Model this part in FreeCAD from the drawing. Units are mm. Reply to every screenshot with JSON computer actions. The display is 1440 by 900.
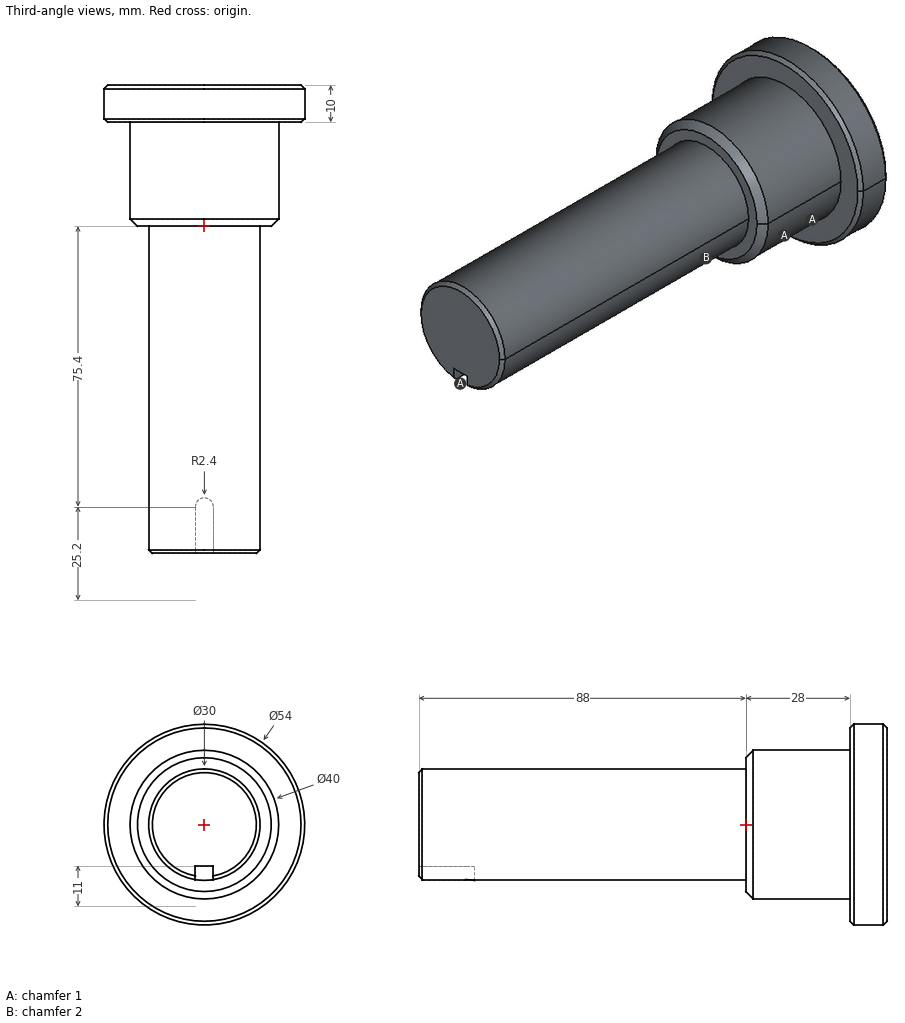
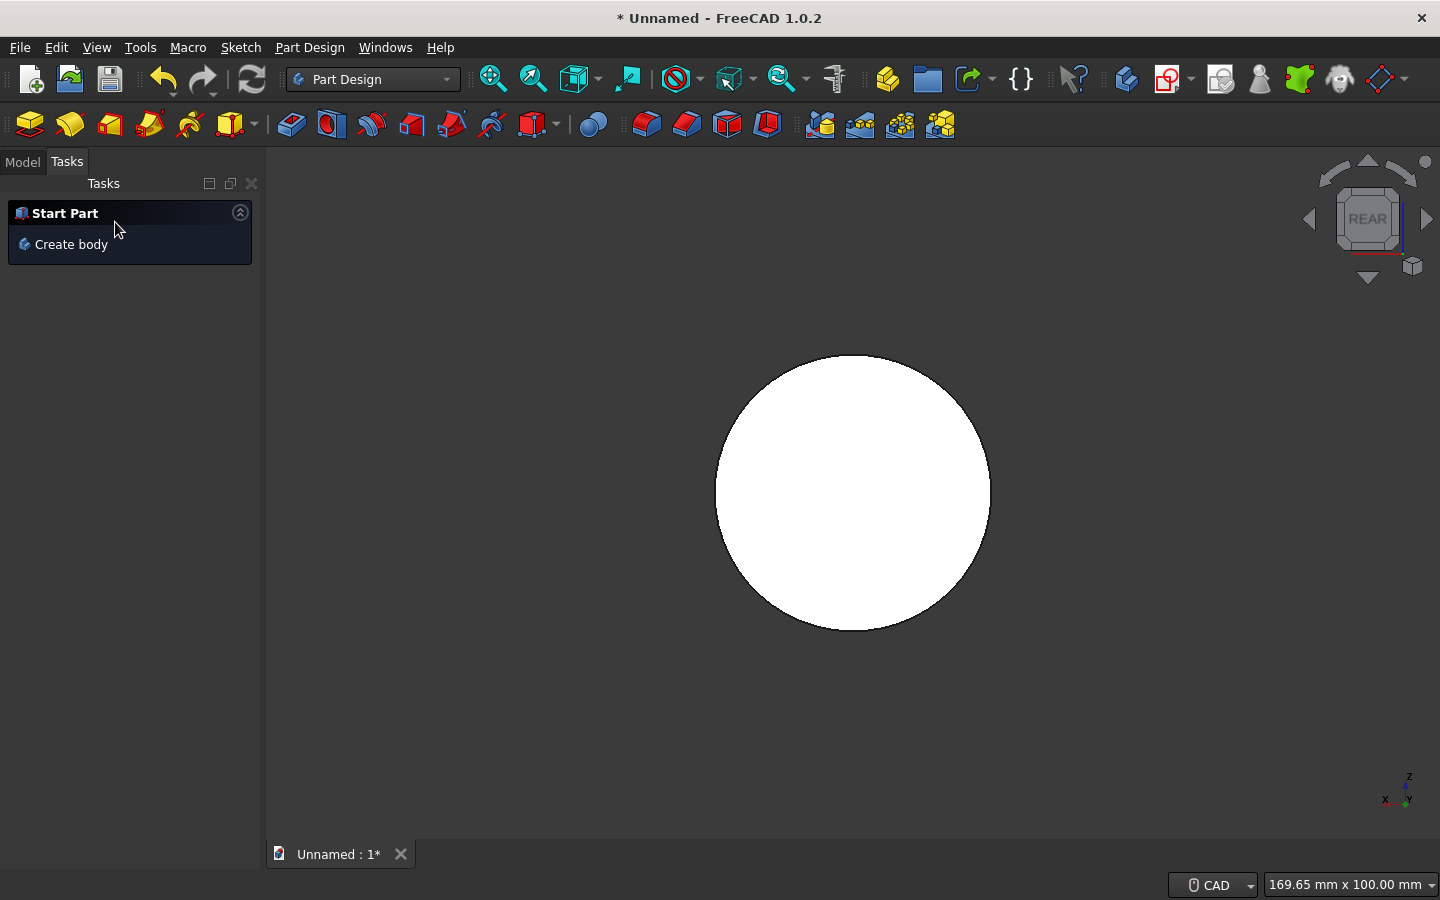
{"action": "key", "text": "v f"}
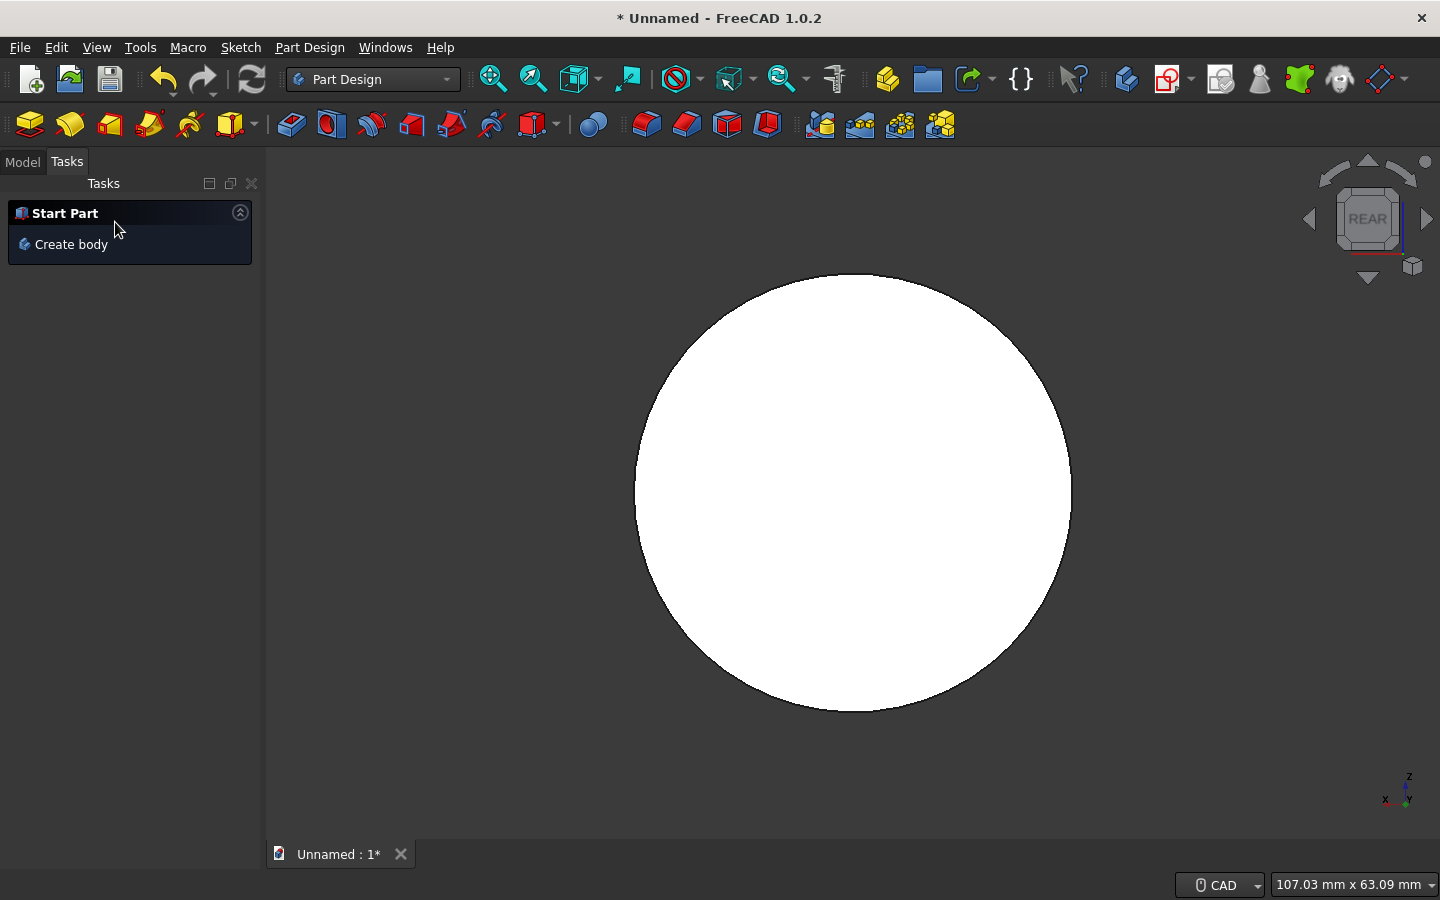
{"action": "left_click", "coordinate": [853, 492]}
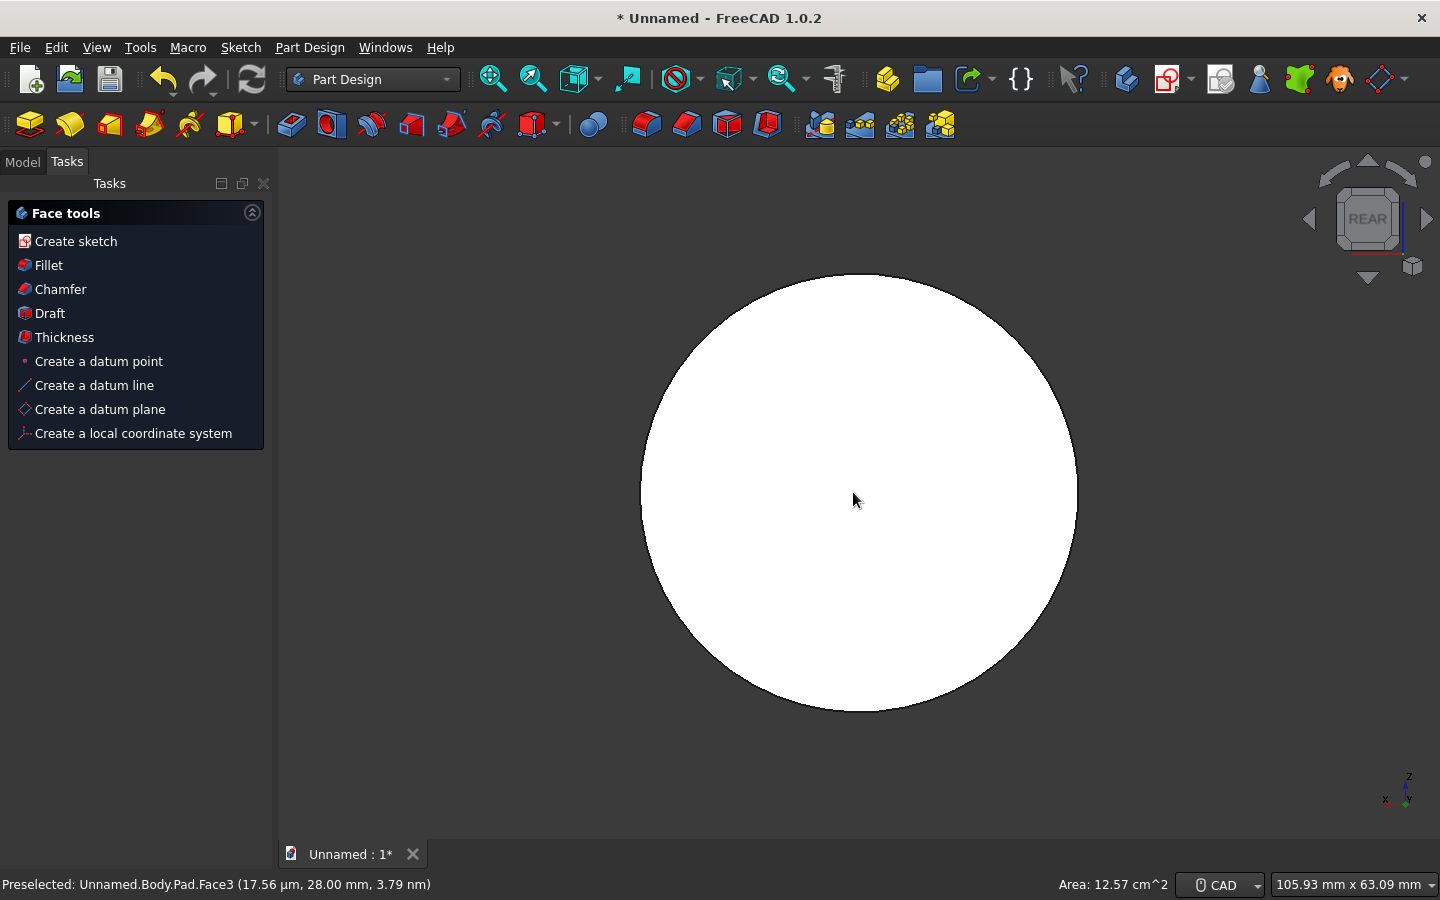
{"action": "left_click", "coordinate": [1168, 80]}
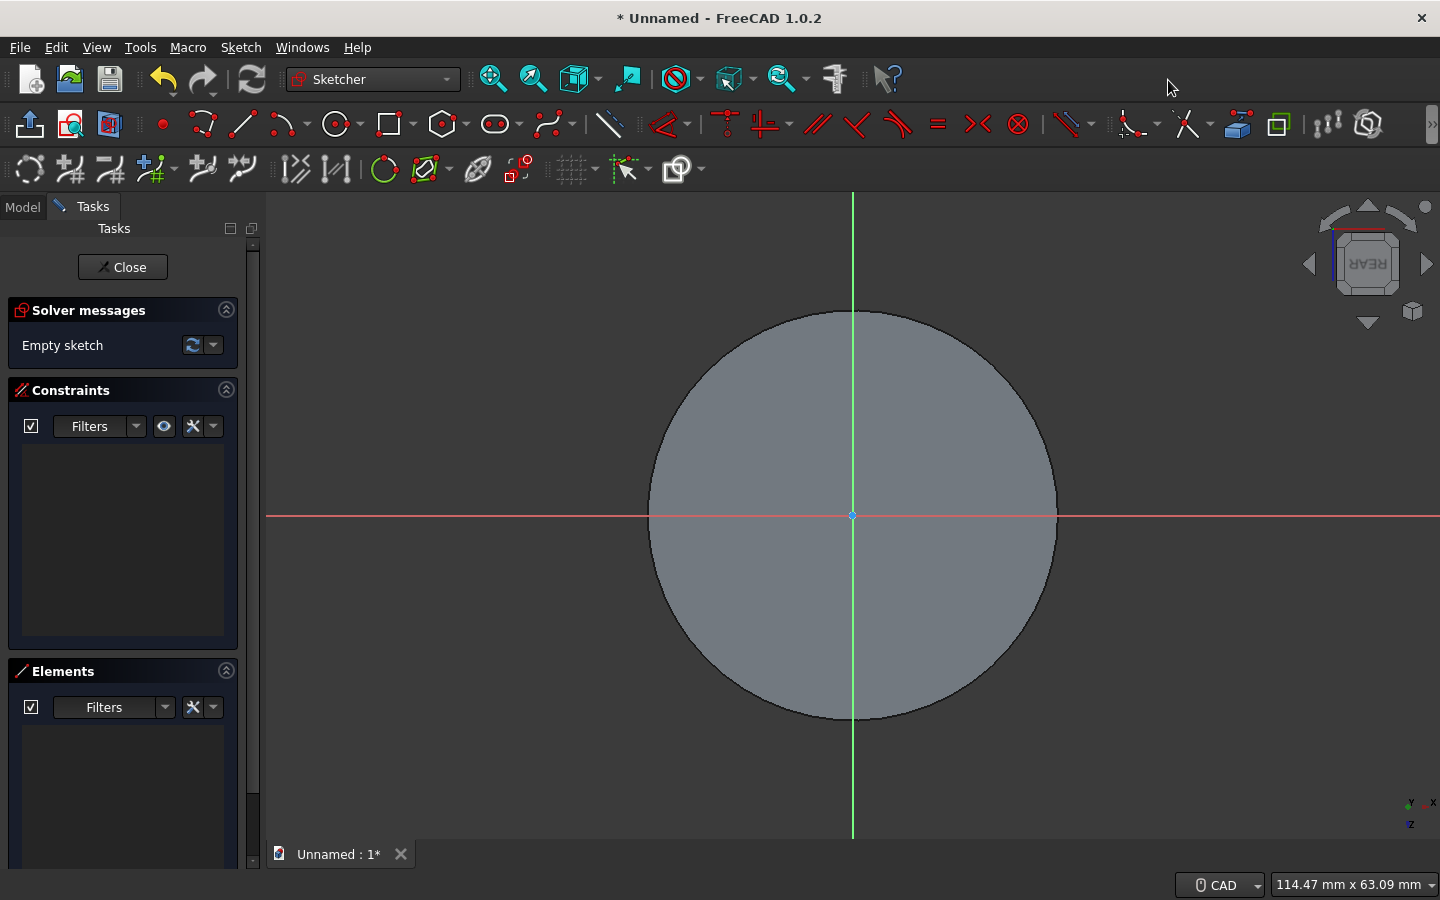
{"action": "scroll", "coordinate": [476, 516], "scroll_direction": "down", "scroll_amount": 1}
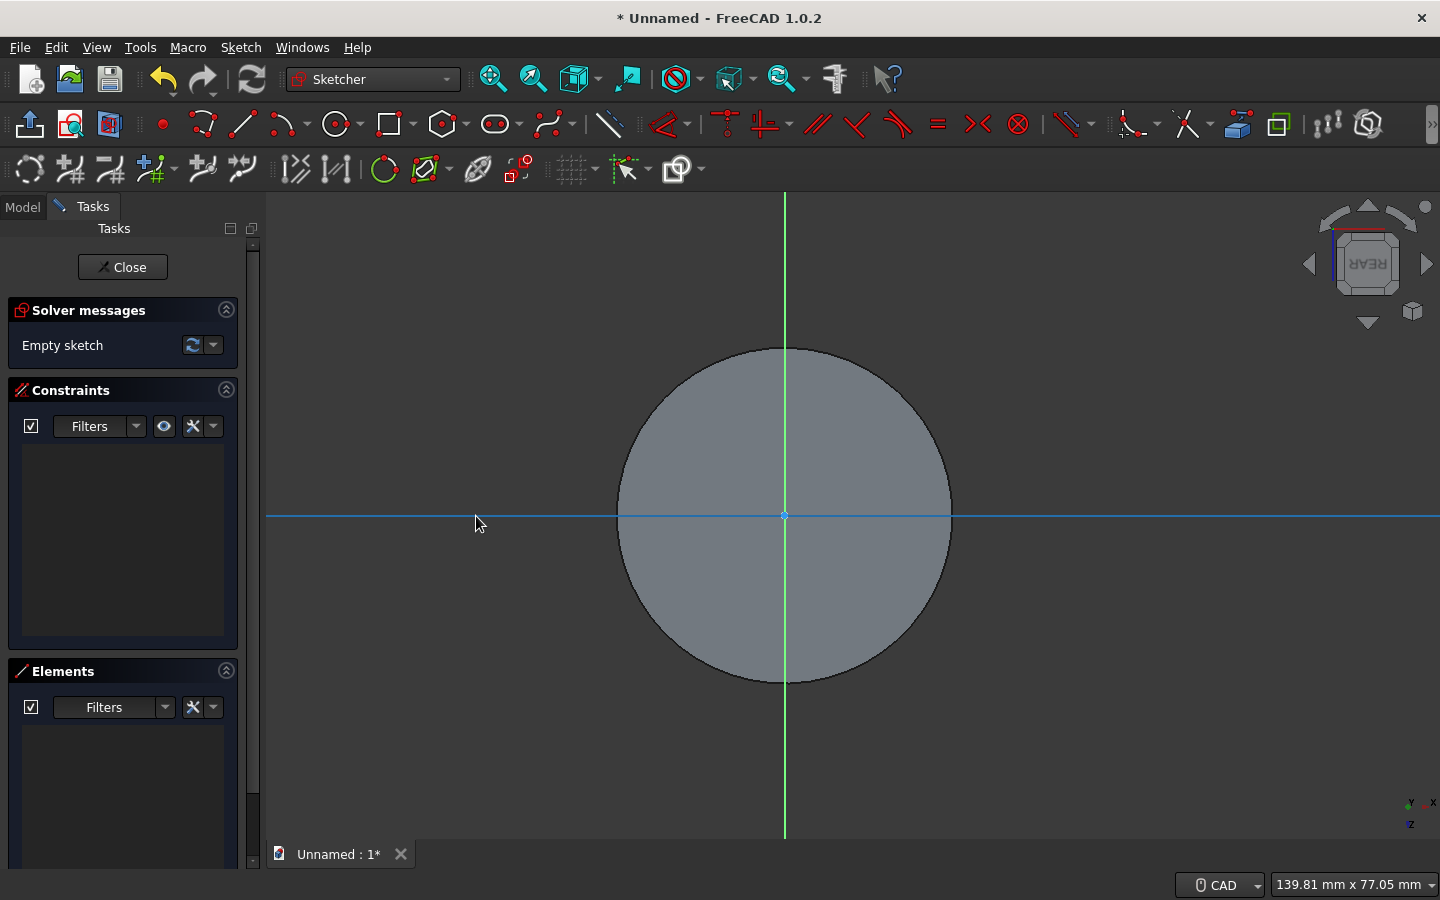
{"action": "key", "text": "g c"}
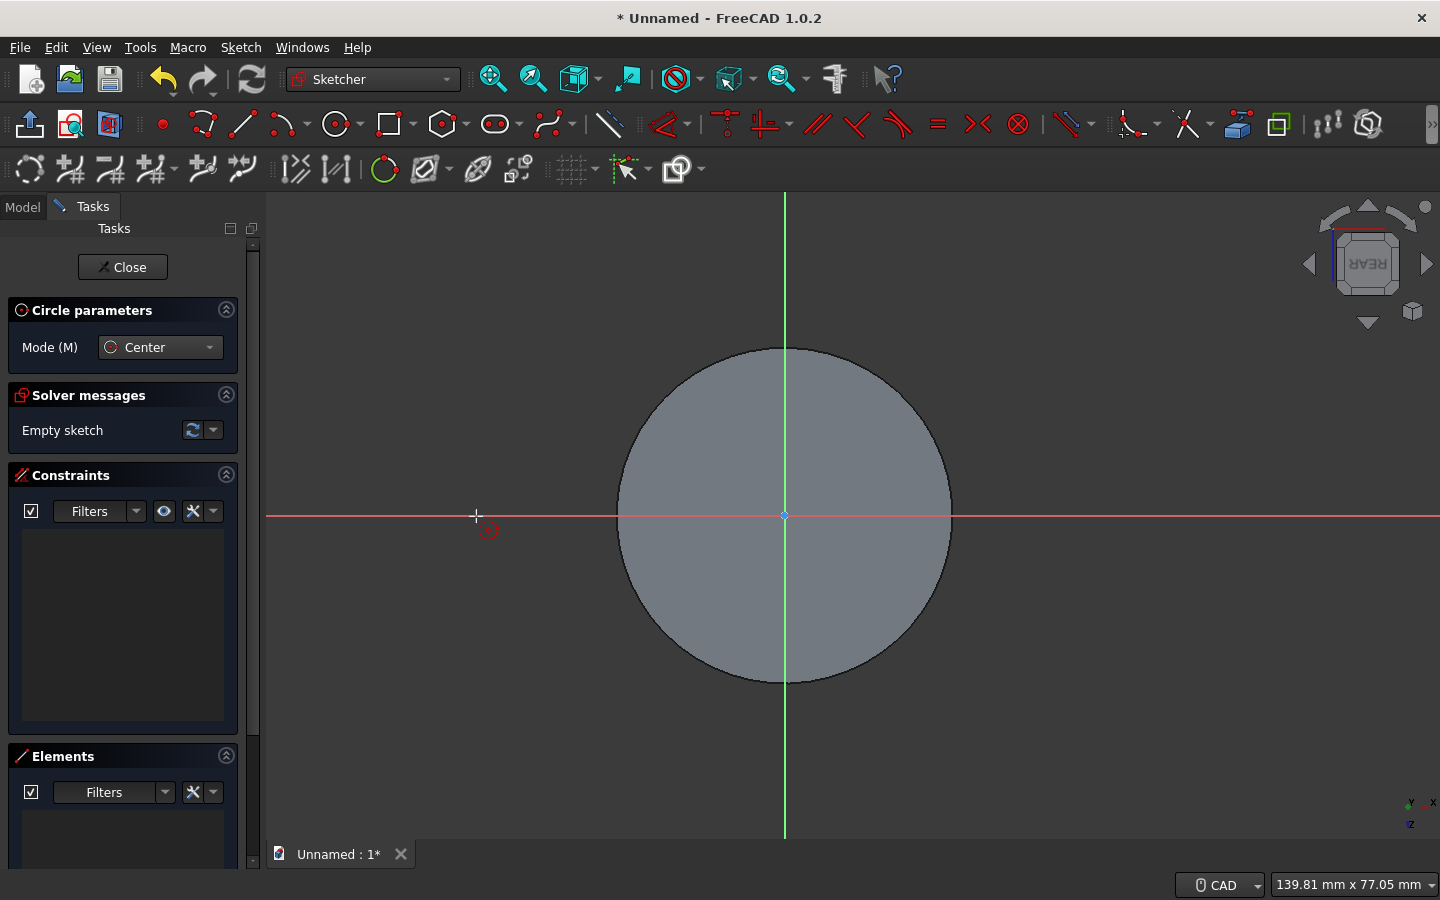
{"action": "left_click", "coordinate": [785, 516]}
{"action": "mouse_move", "coordinate": [945, 355]}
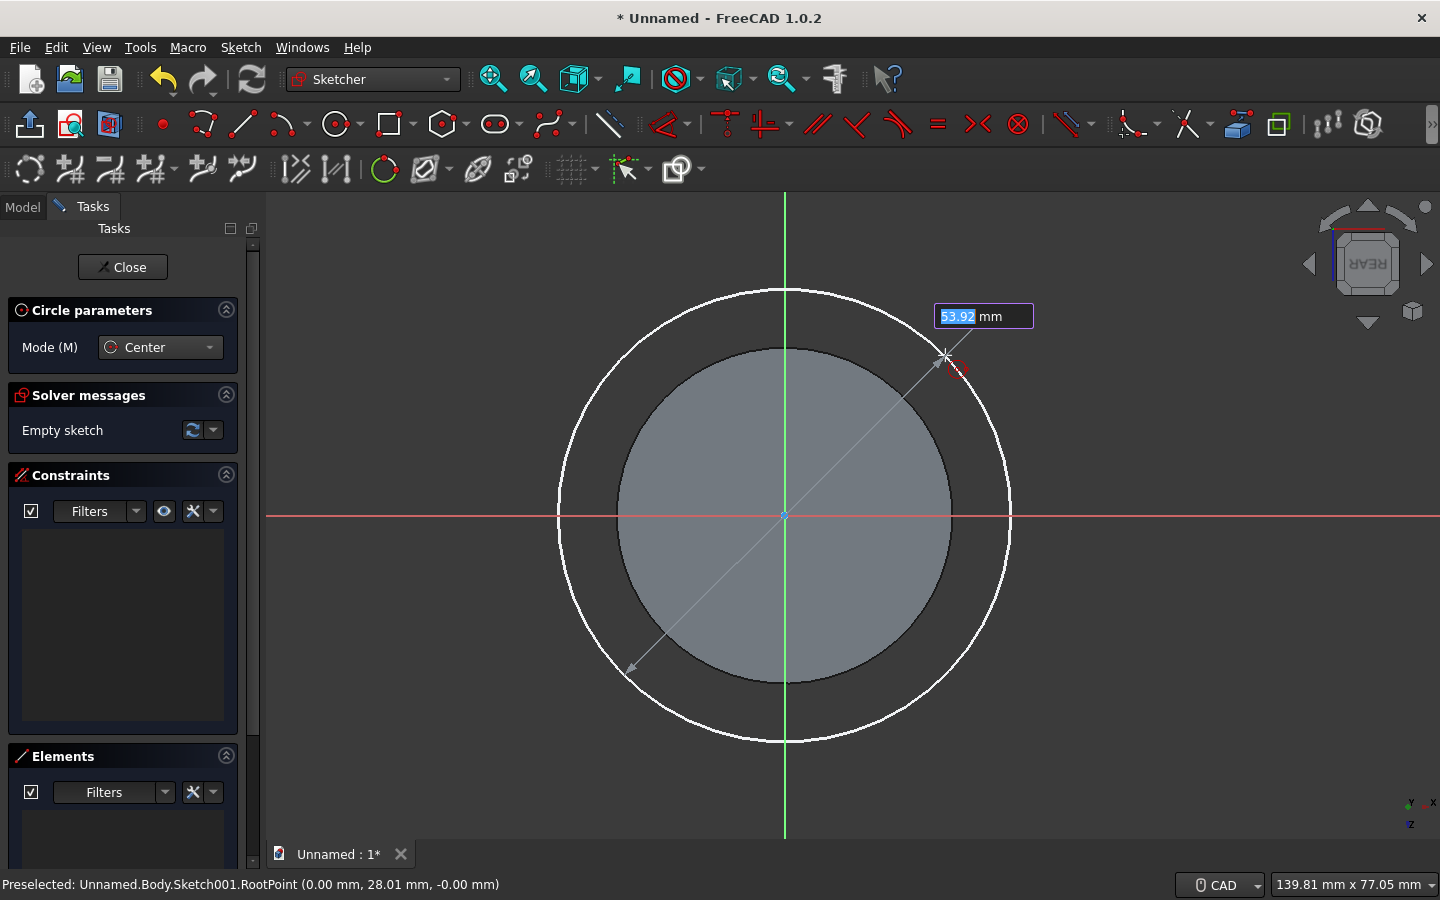
{"action": "type", "text": "54"}
{"action": "key", "text": "Return"}
{"action": "key", "text": "Escape"}